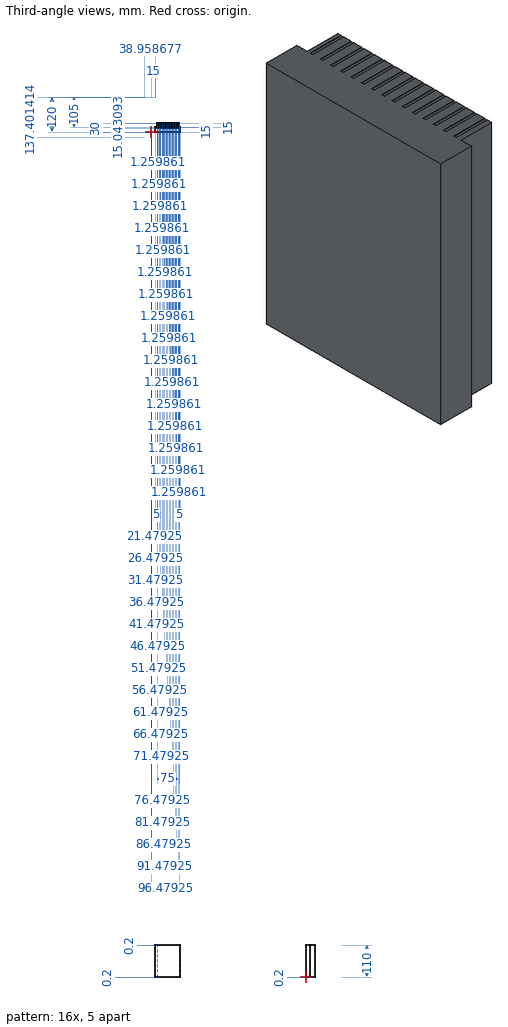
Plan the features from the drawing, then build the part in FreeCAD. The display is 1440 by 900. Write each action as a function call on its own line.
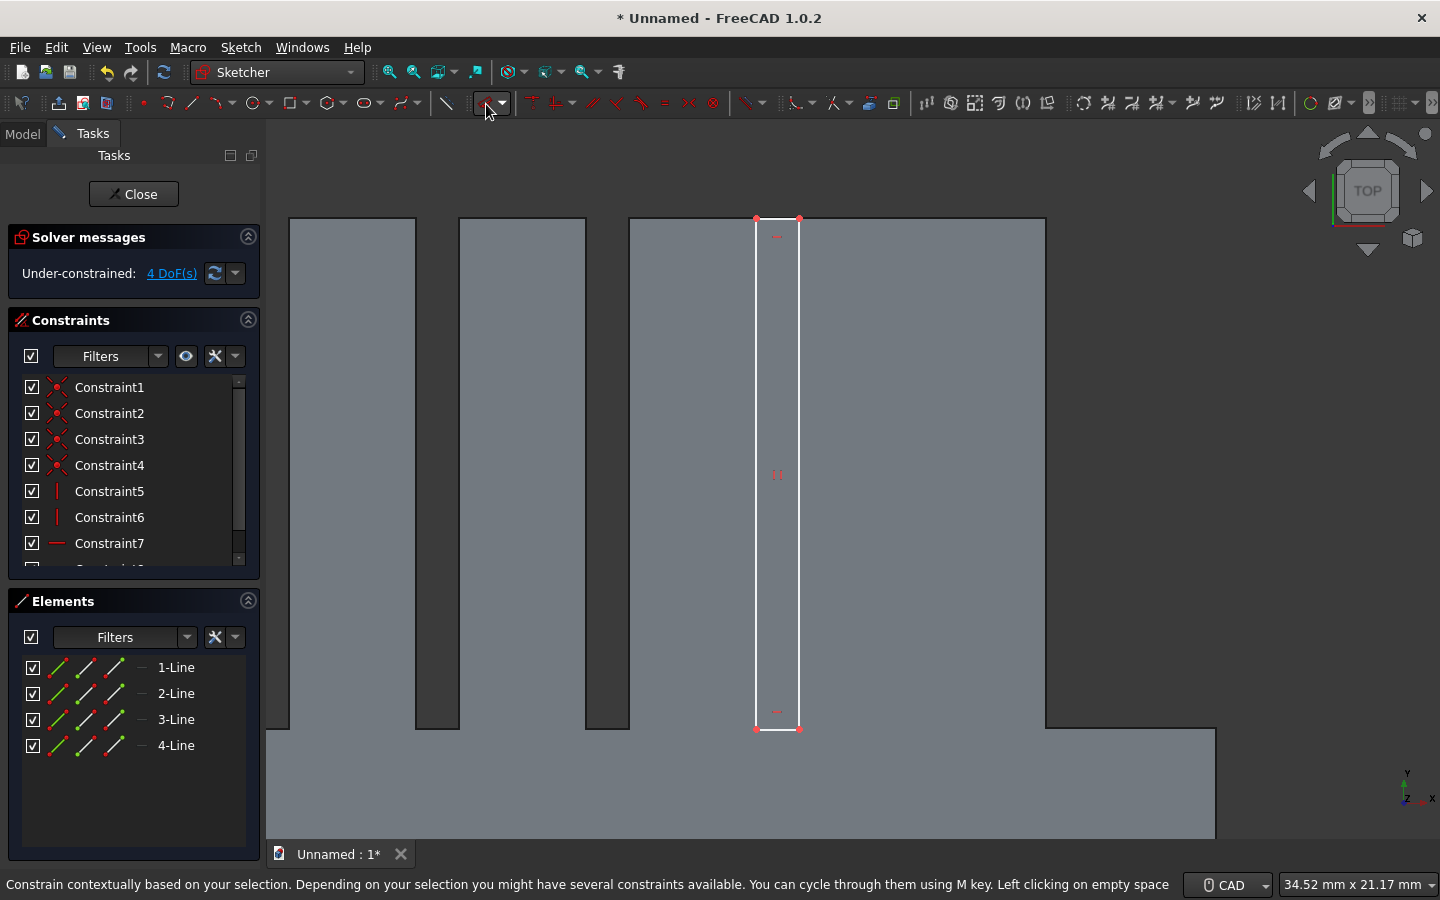
click(756, 219)
click(814, 515)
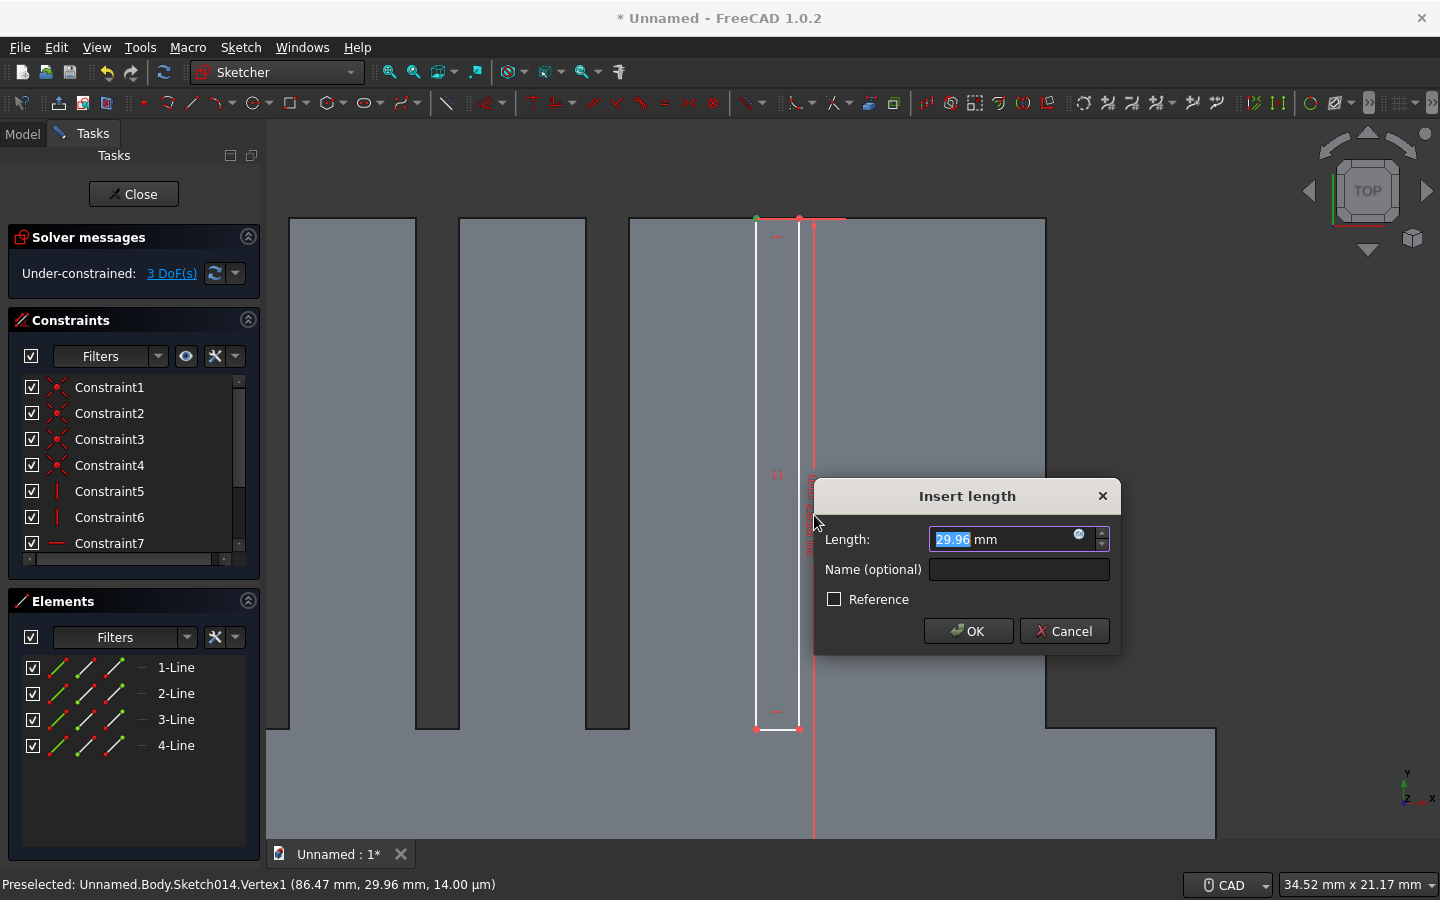
text(30)
key(Return)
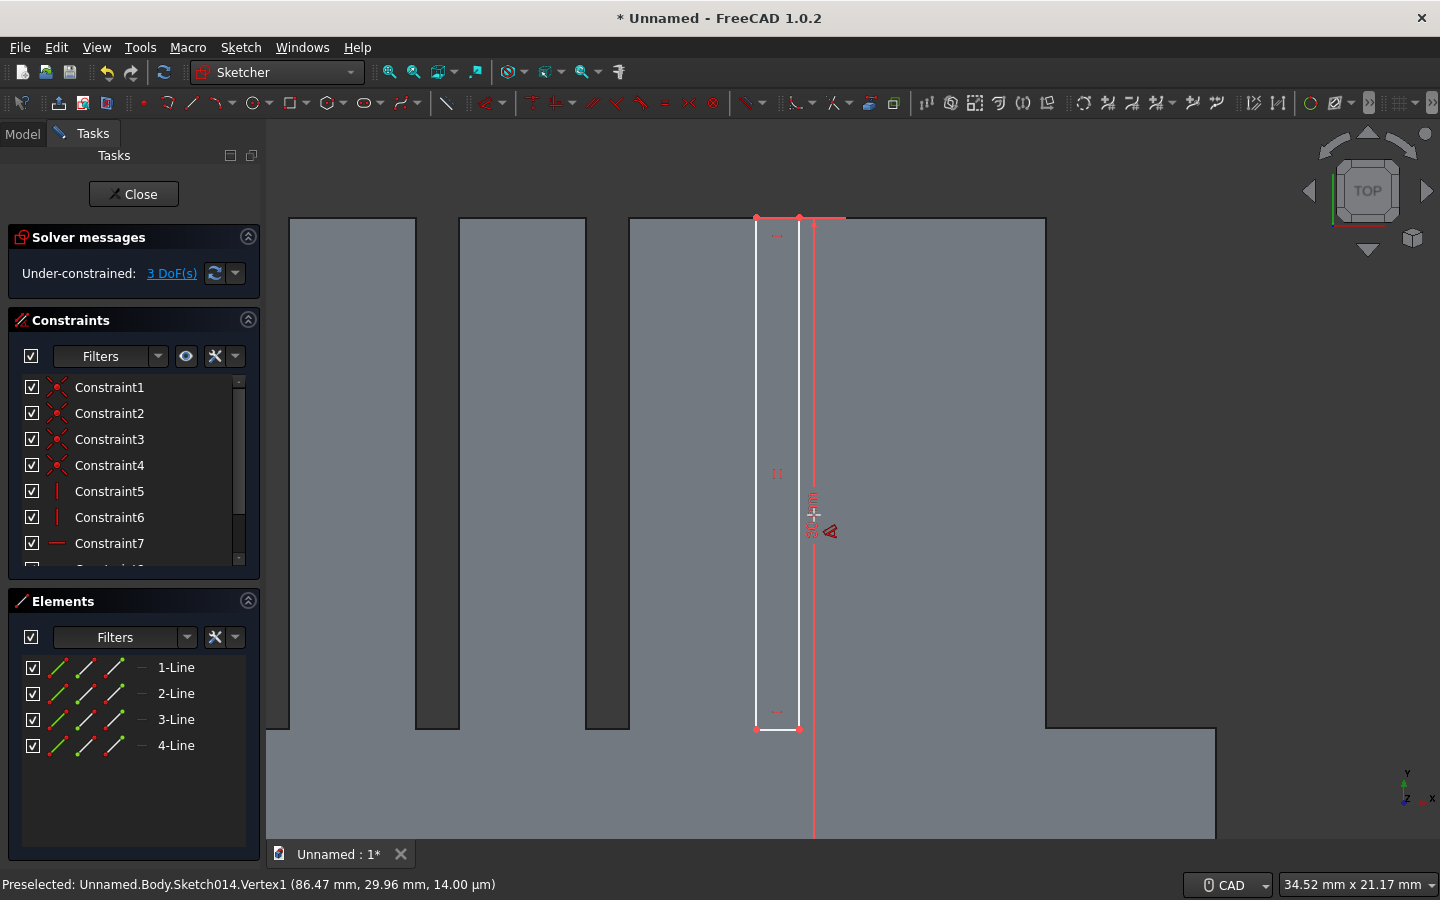
click(769, 730)
click(778, 764)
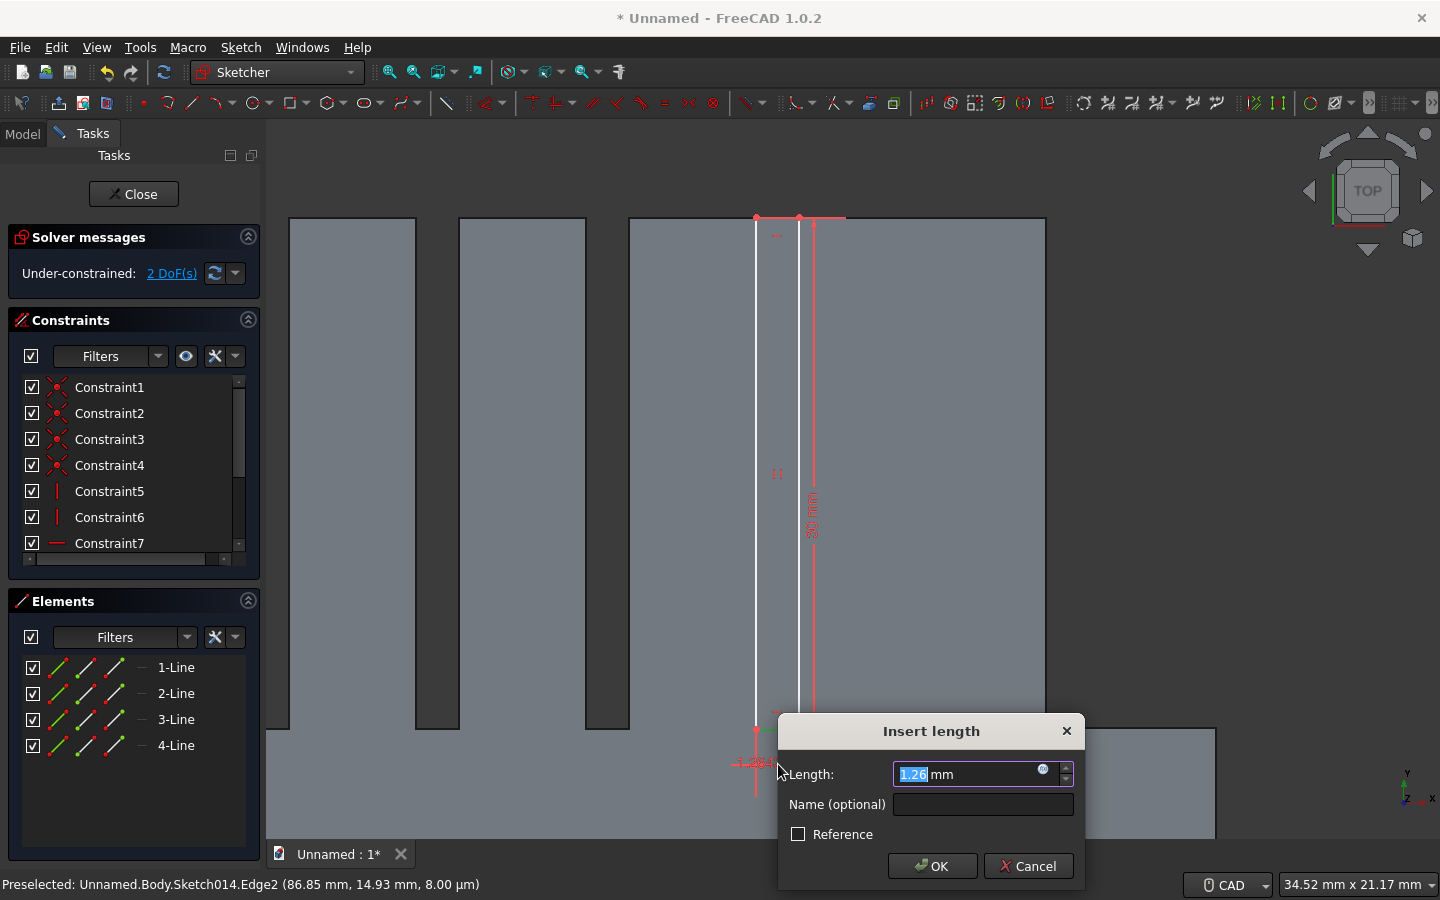
text(1.259861)
key(Return)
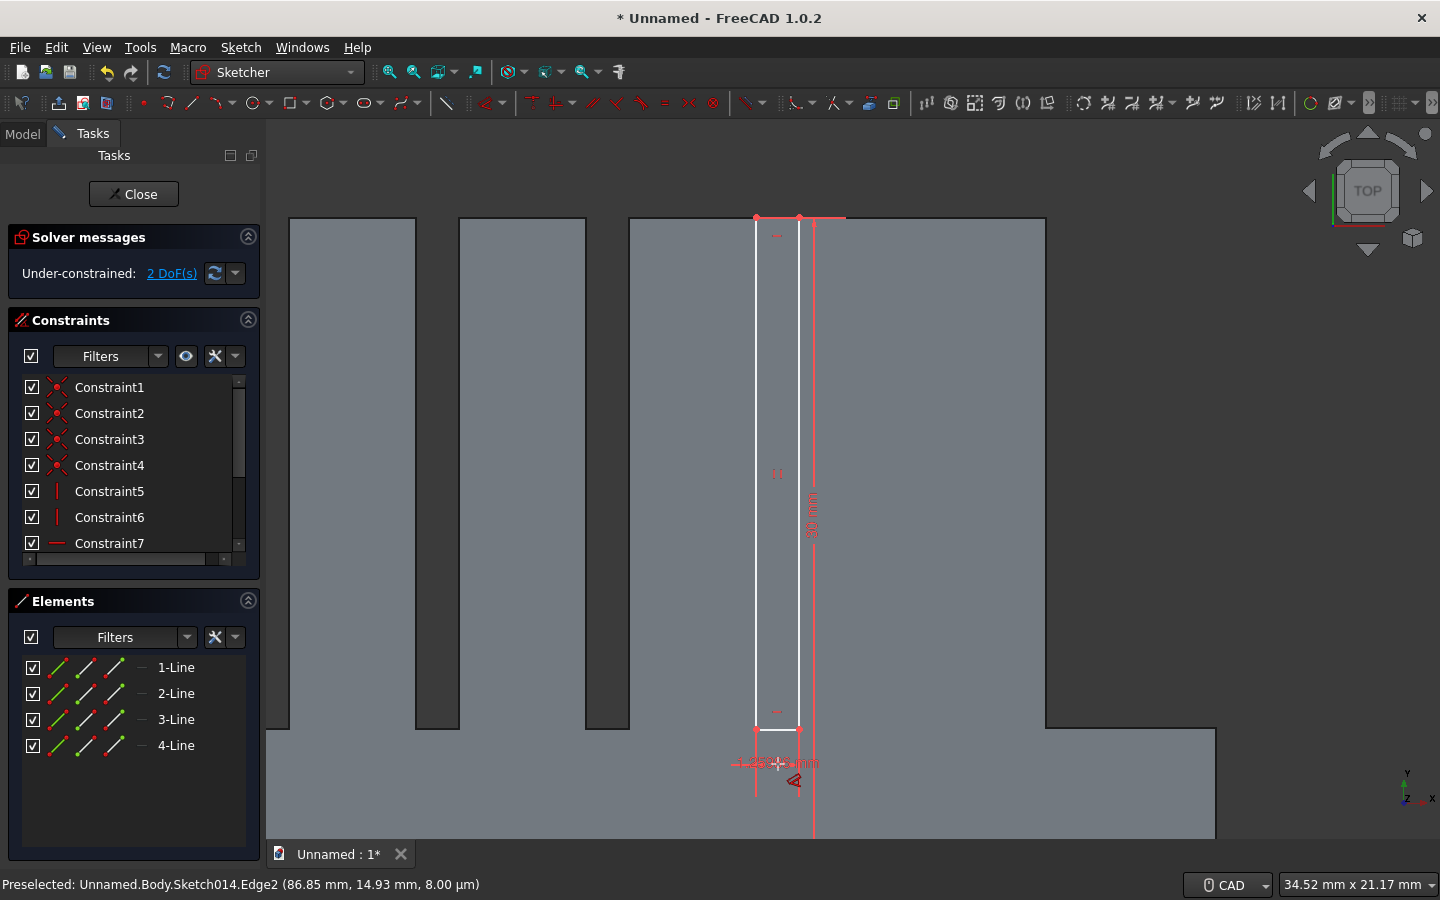
click(756, 371)
click(722, 474)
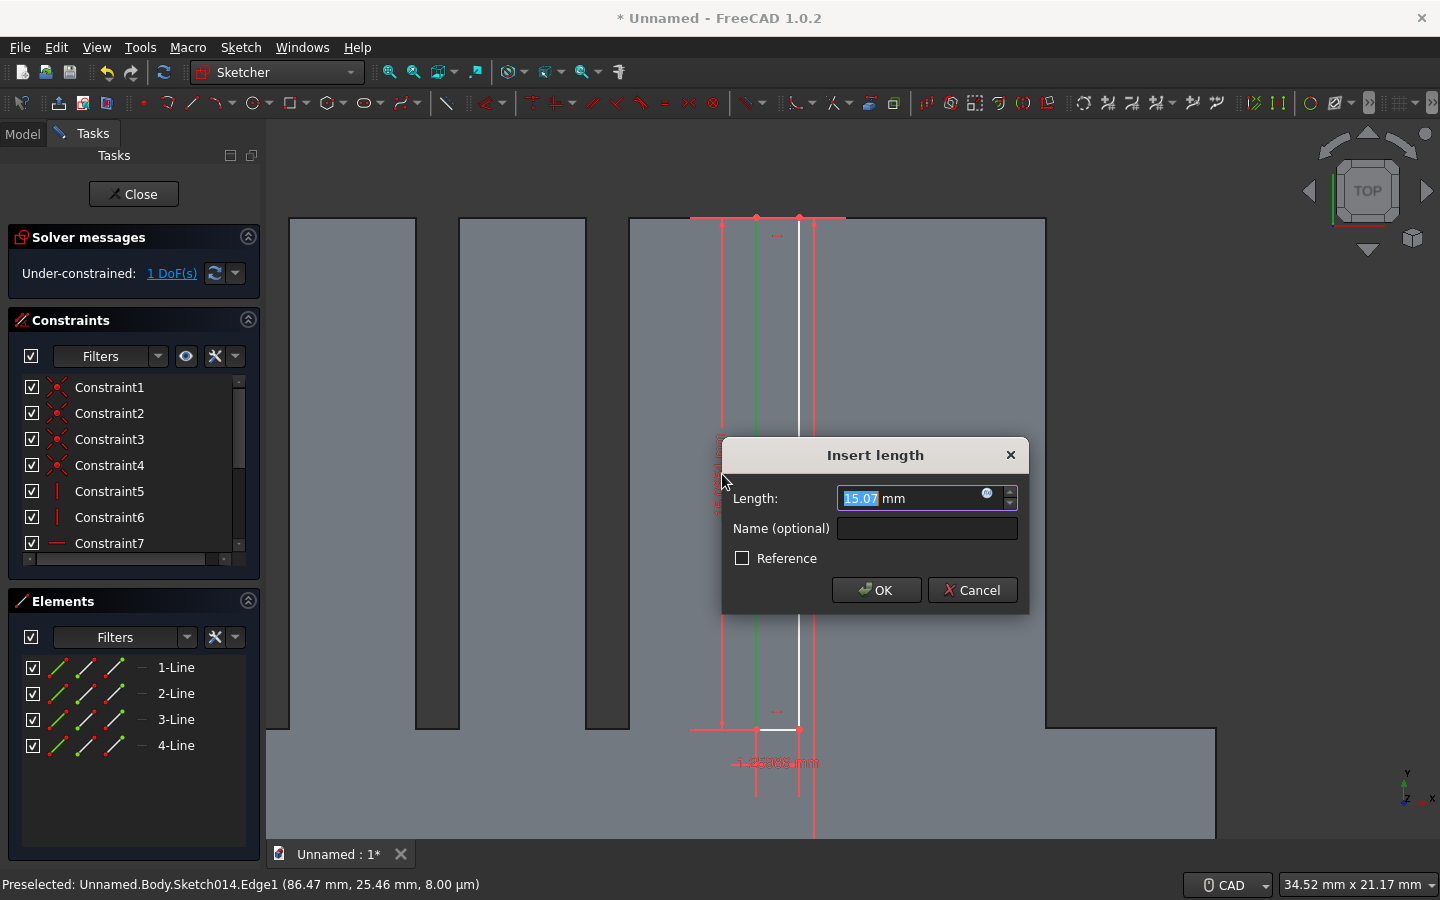
text(15.043093)
key(Return)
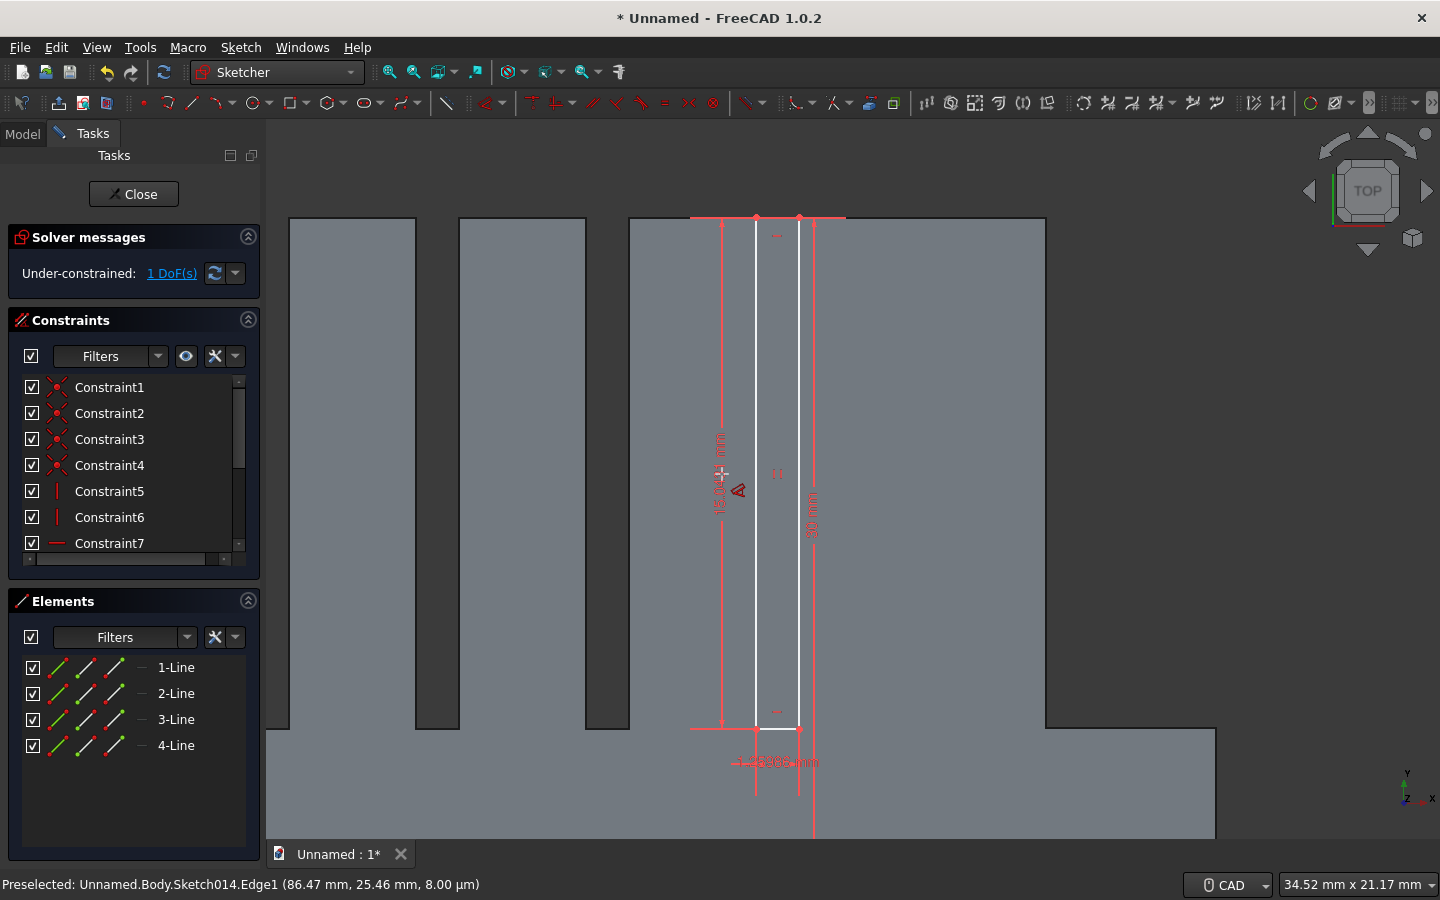
click(756, 218)
click(525, 184)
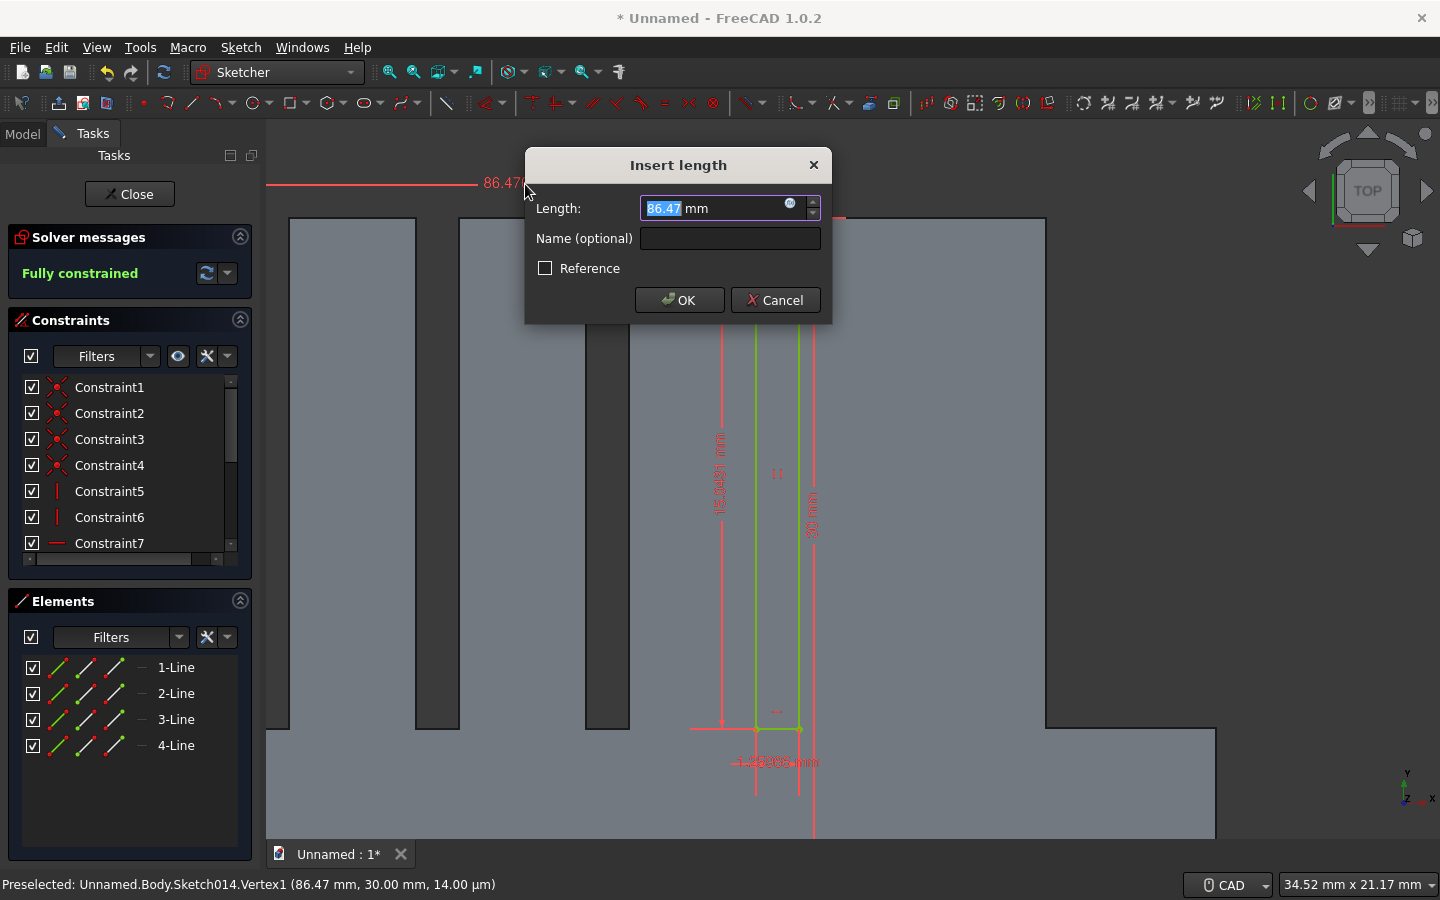
text(86.47925)
key(Return)
key(Escape)